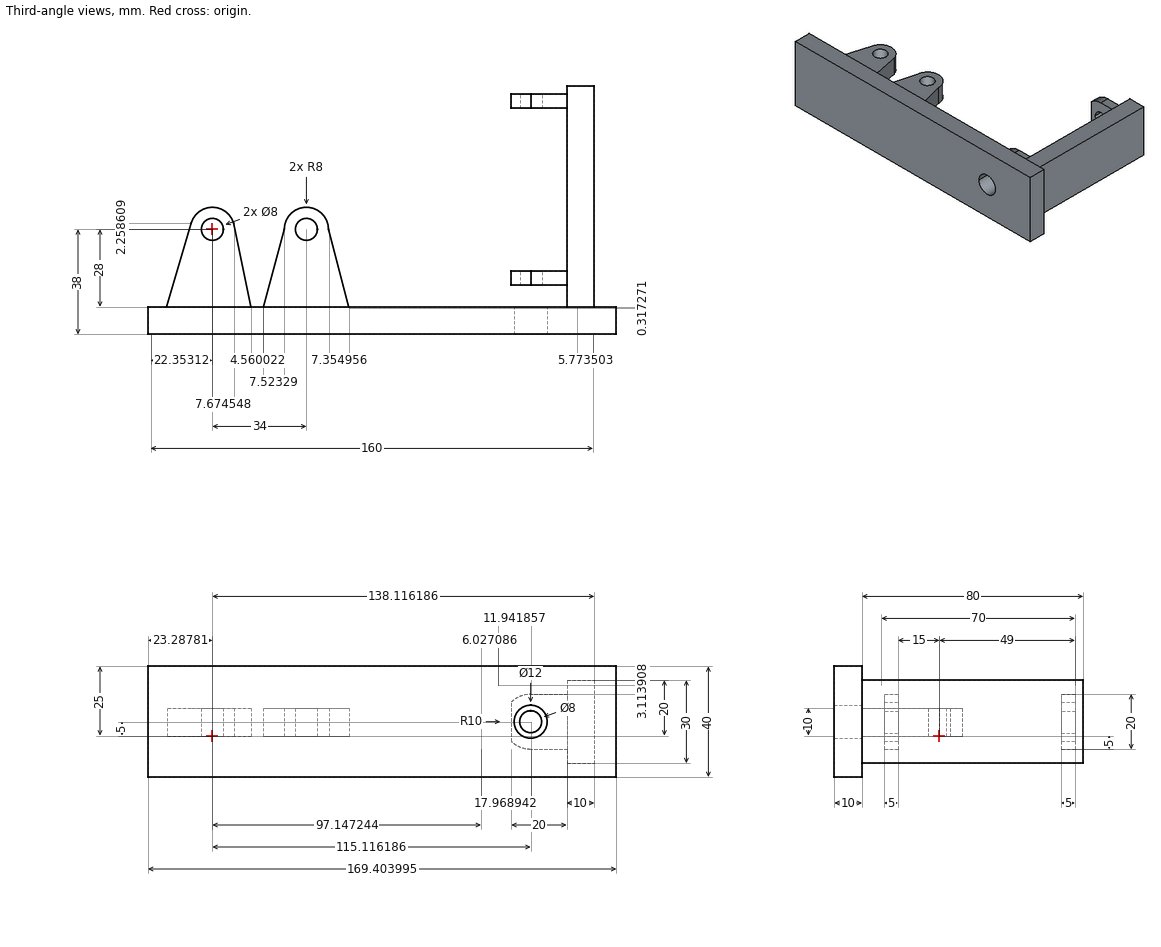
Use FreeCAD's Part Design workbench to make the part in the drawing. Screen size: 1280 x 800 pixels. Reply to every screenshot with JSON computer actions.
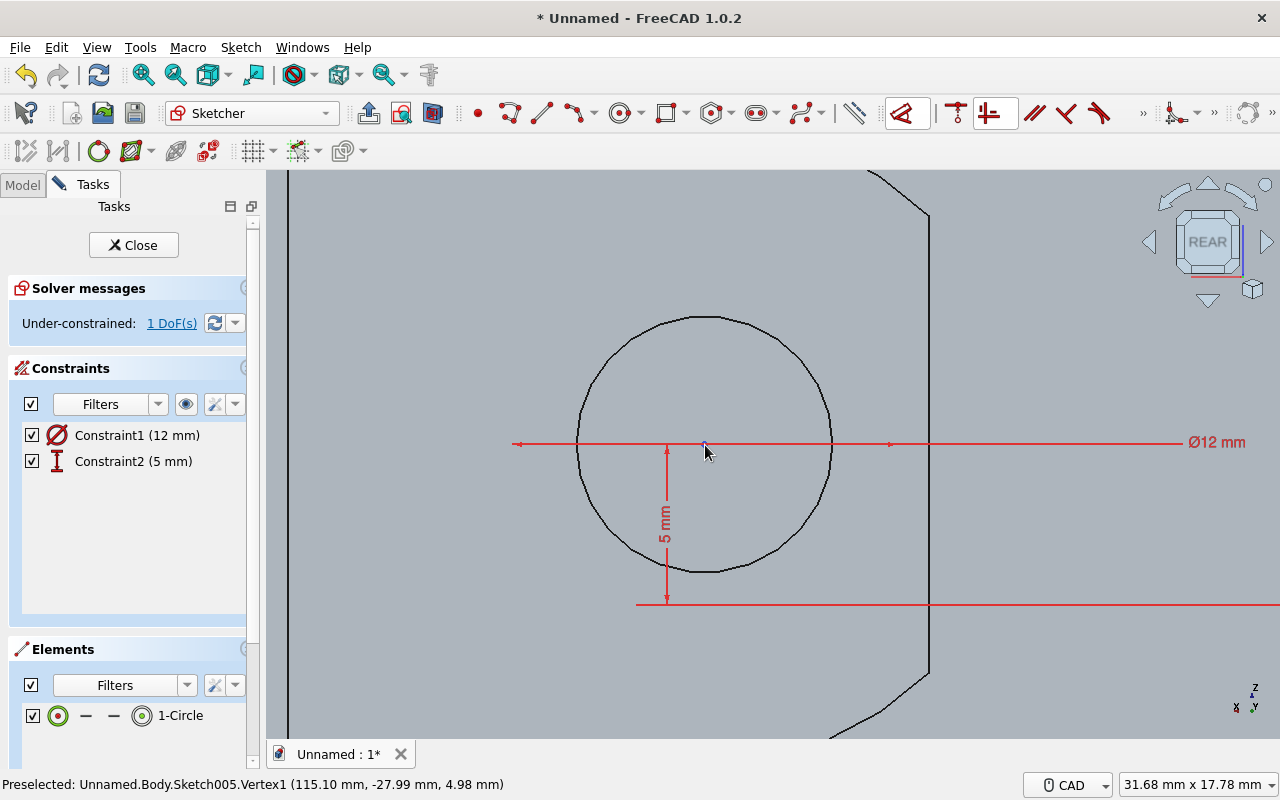
{"action": "left_click", "coordinate": [705, 444]}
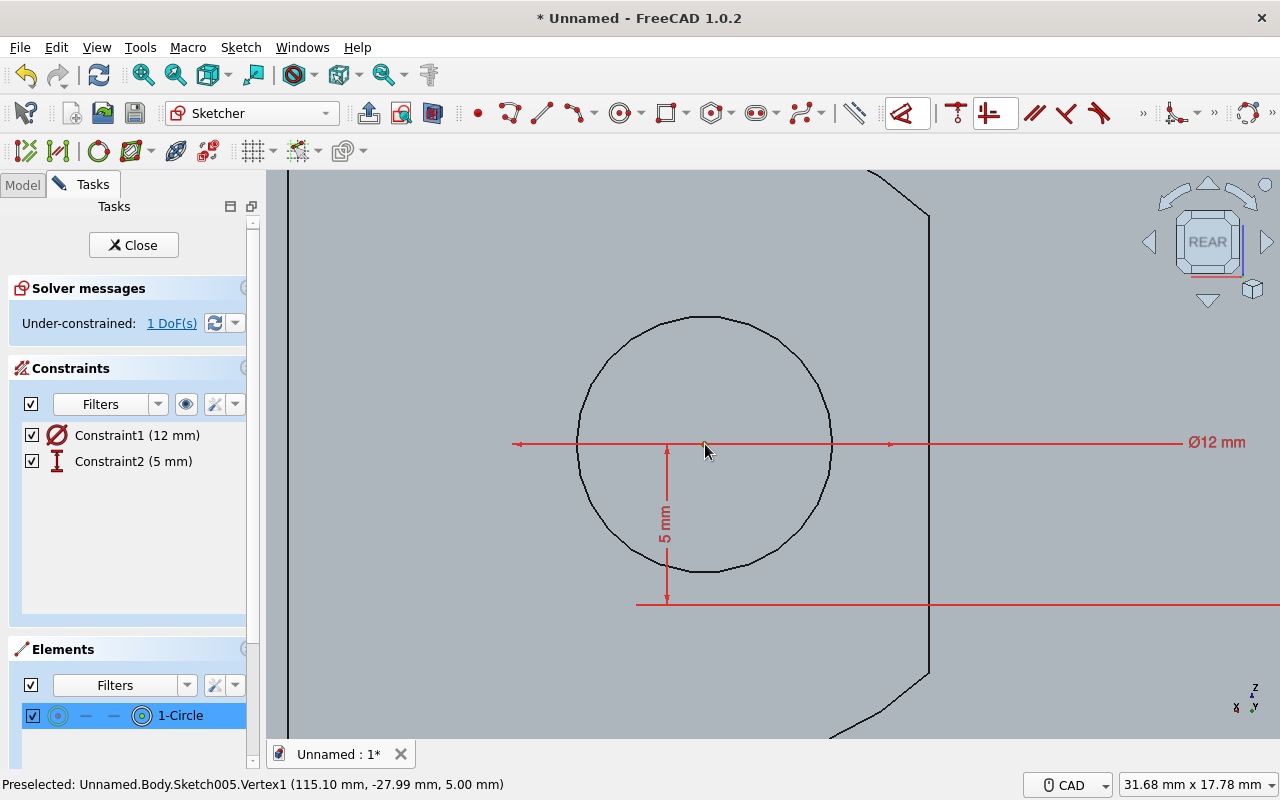
{"action": "key", "text": "l"}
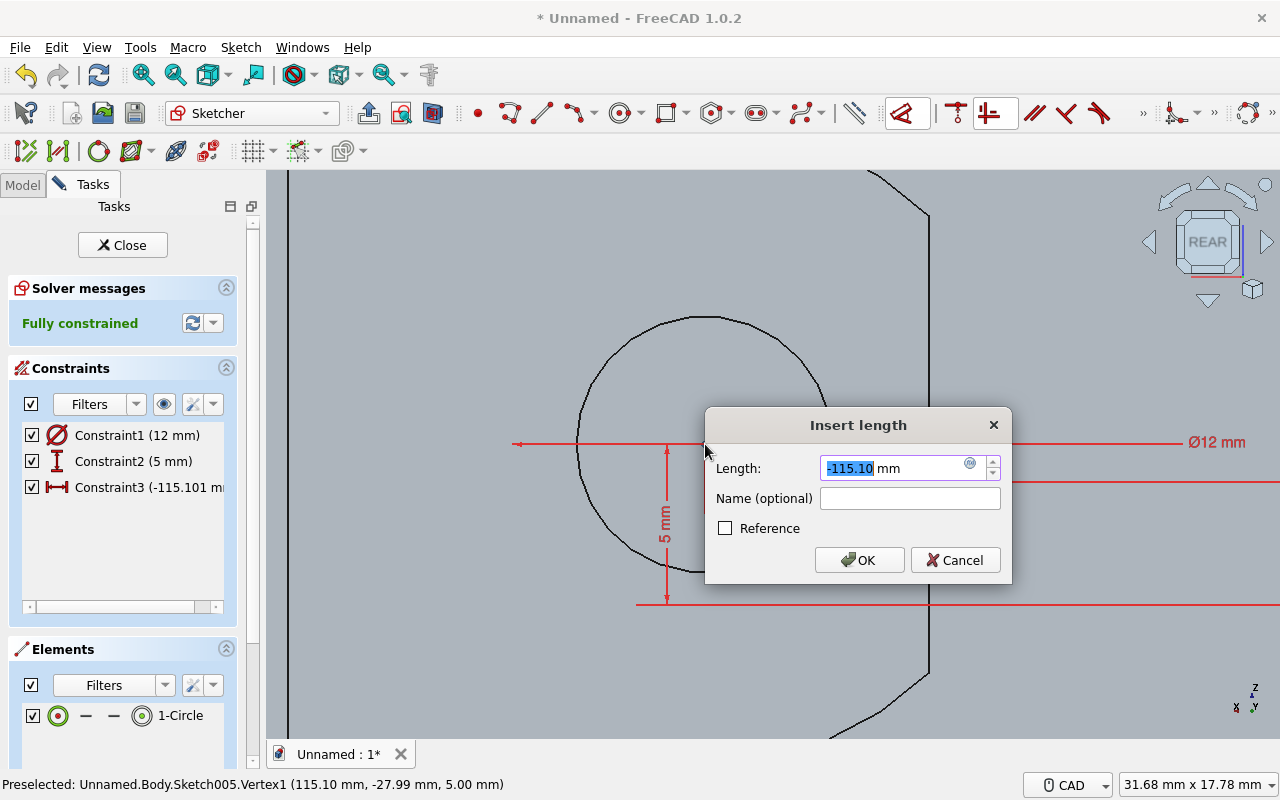
{"action": "type", "text": "-115.116186"}
{"action": "key", "text": "Return"}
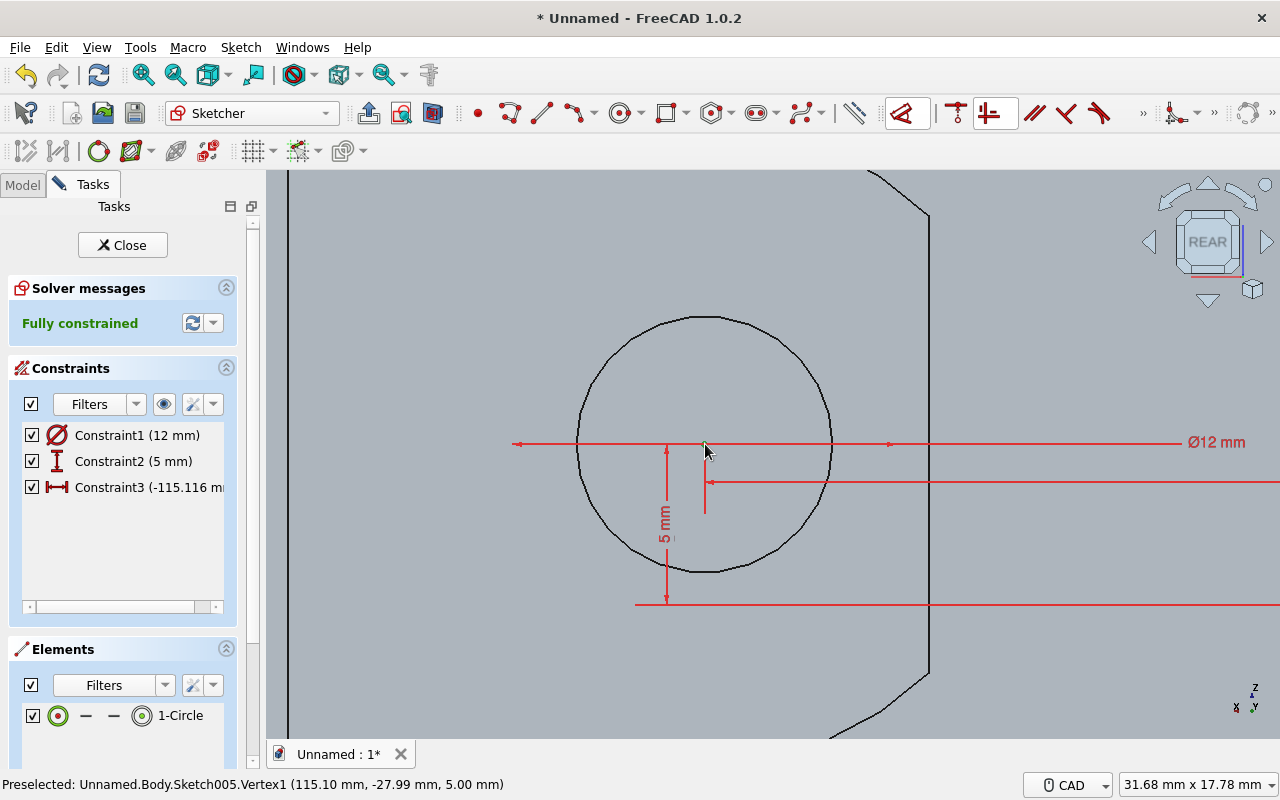
{"action": "left_click", "coordinate": [123, 245]}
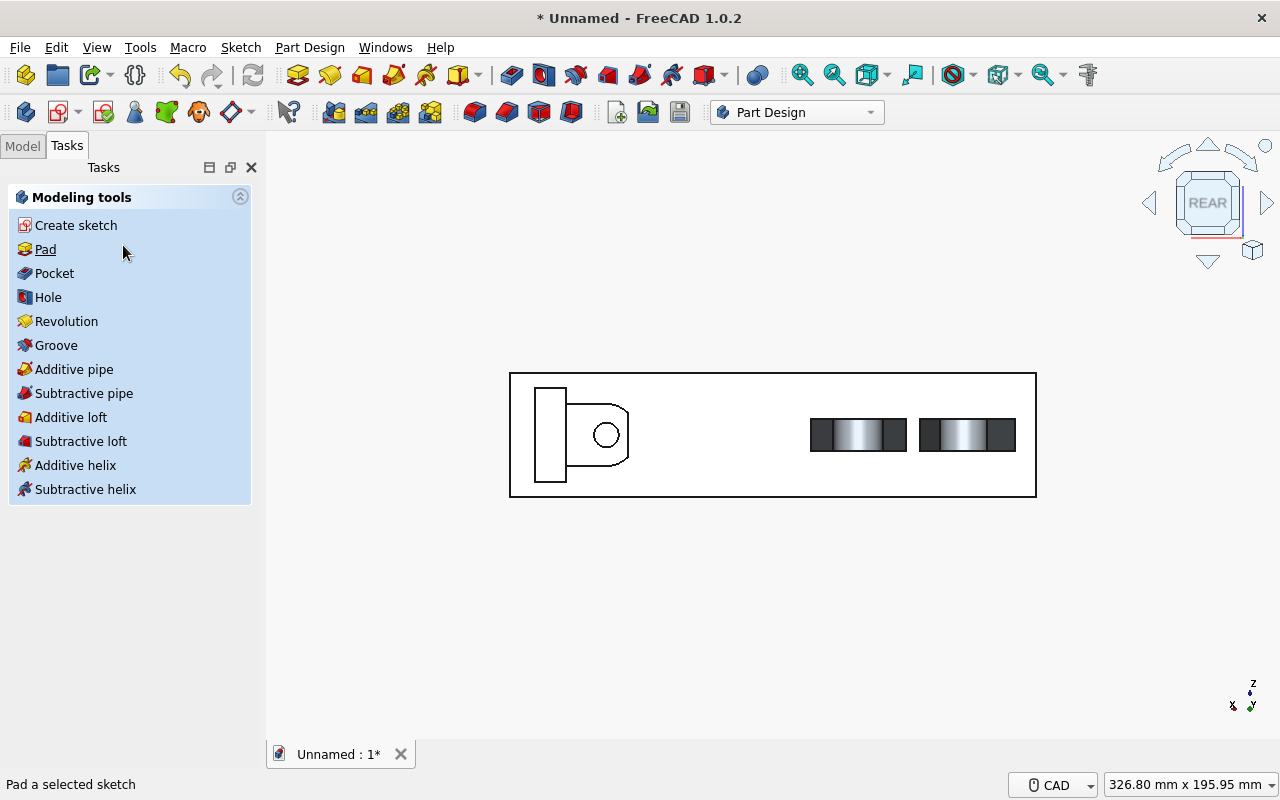
{"action": "left_click", "coordinate": [512, 76]}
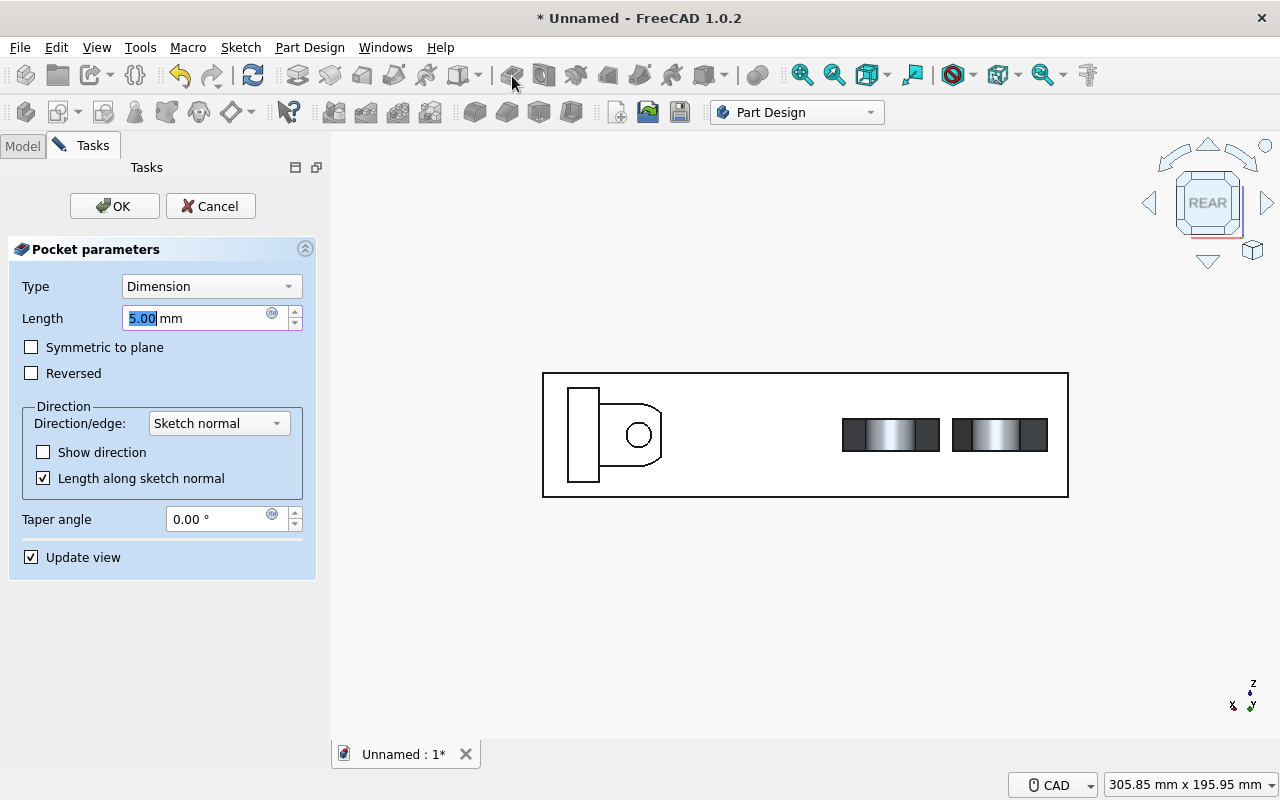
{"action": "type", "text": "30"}
{"action": "key", "text": "Tab"}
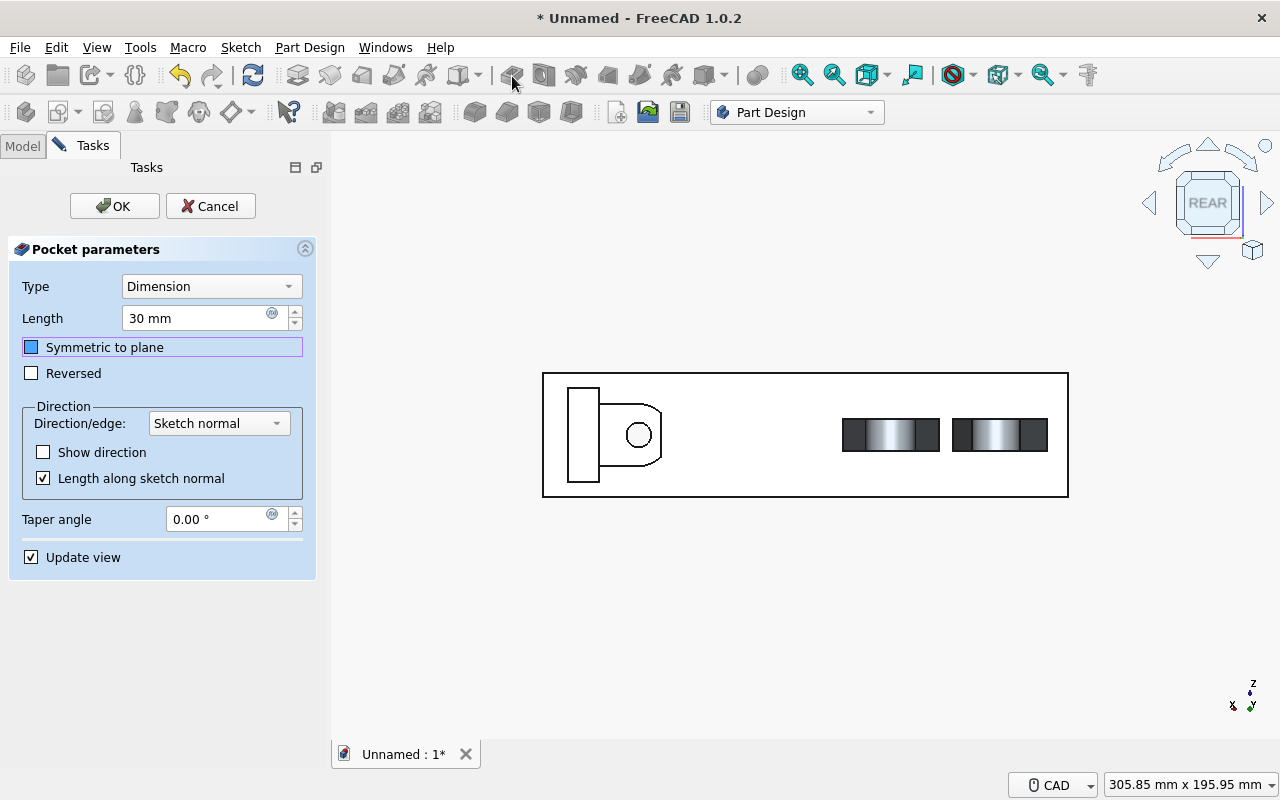
{"action": "left_click", "coordinate": [115, 206]}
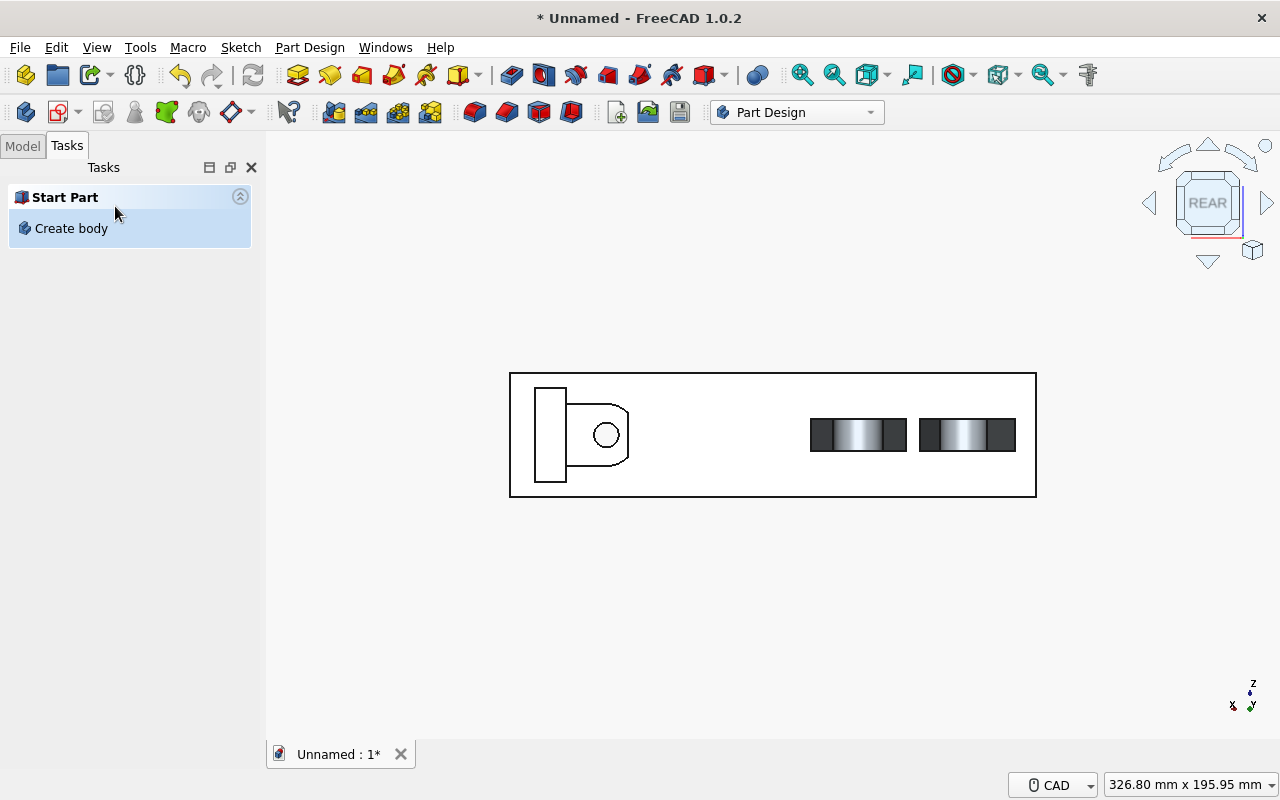
{"action": "key", "text": "0"}